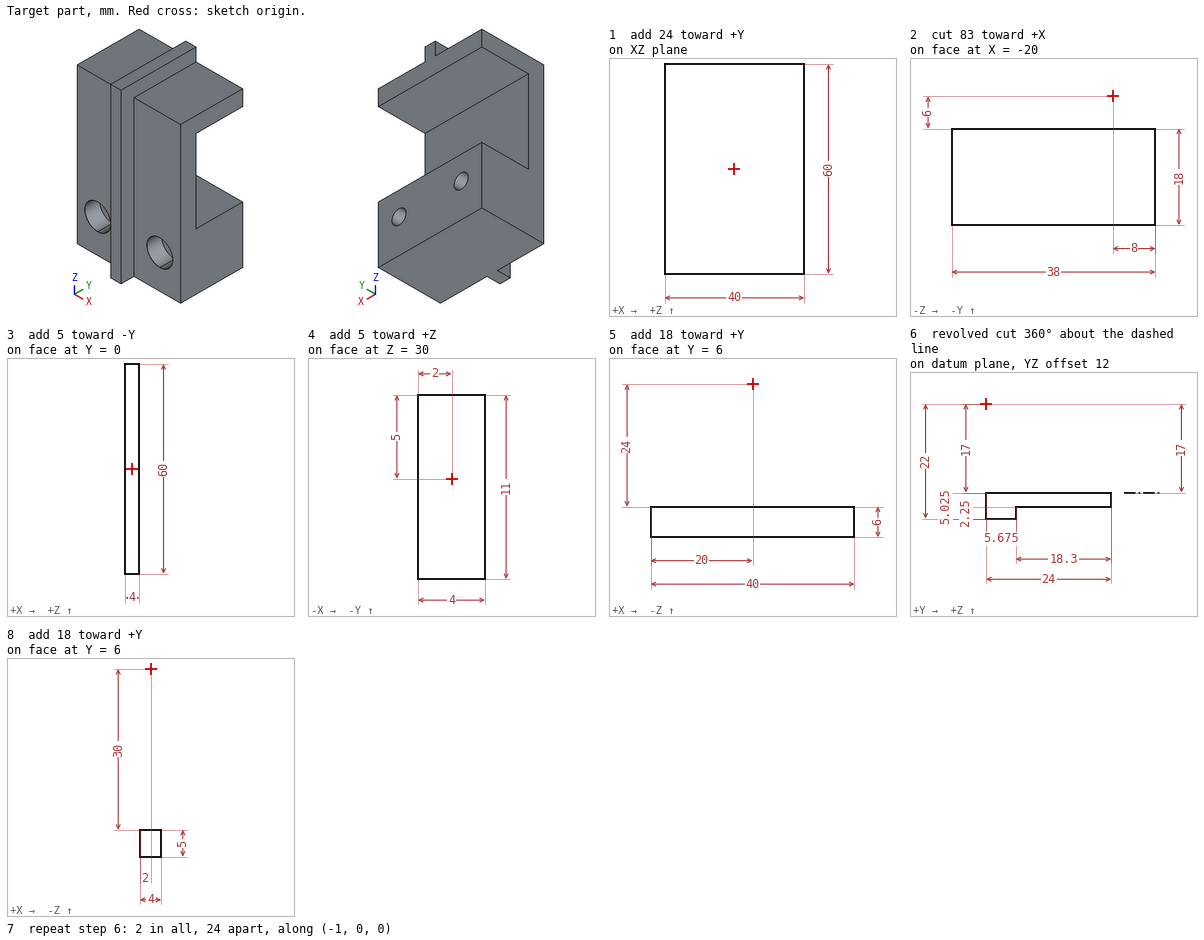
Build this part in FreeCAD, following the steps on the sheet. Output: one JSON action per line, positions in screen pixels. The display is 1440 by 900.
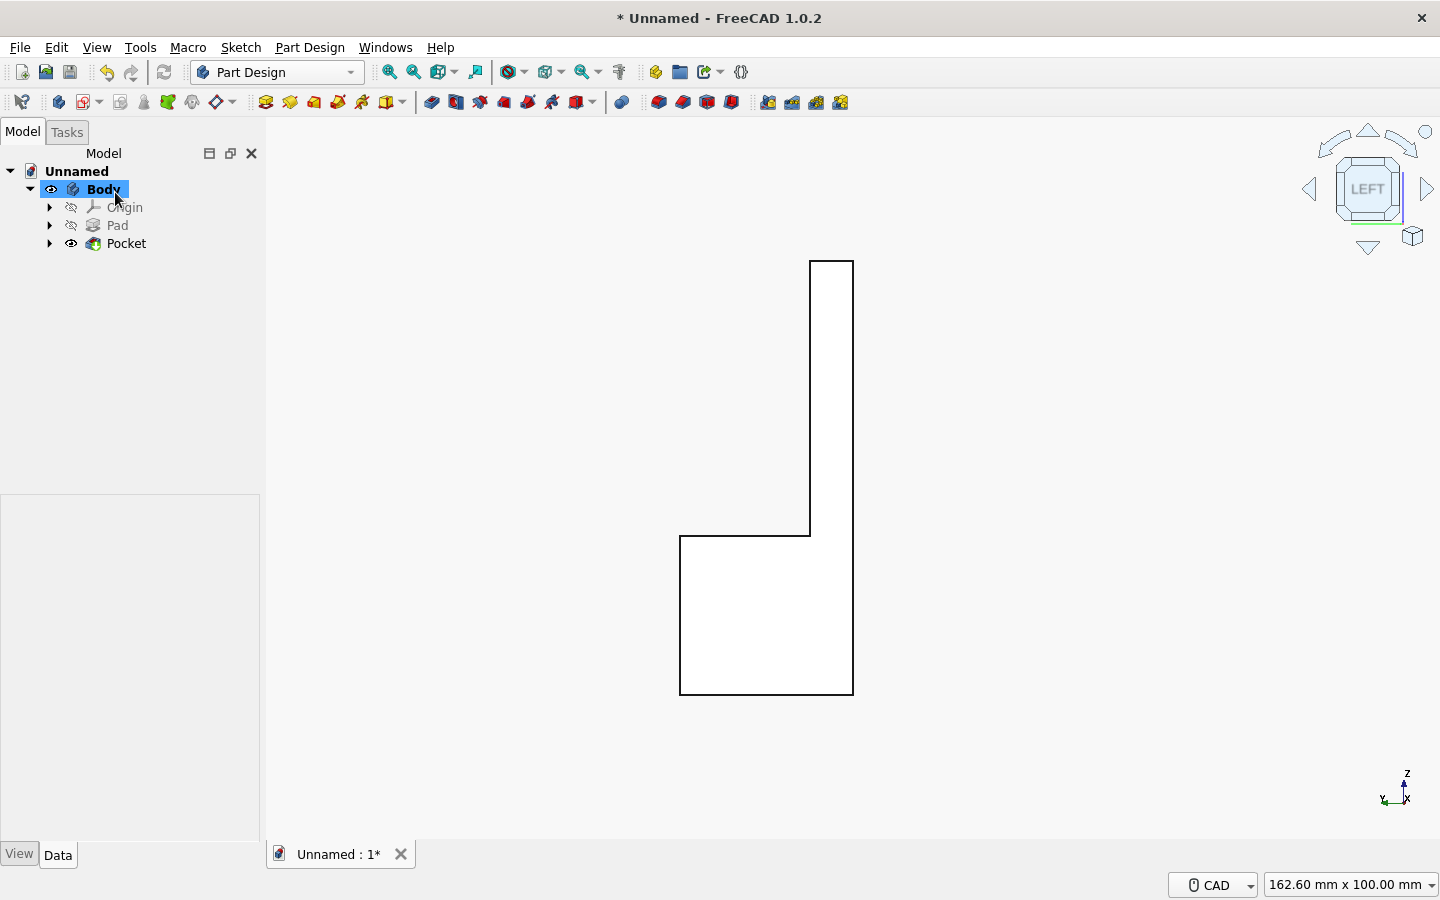
{"action": "key", "text": "0"}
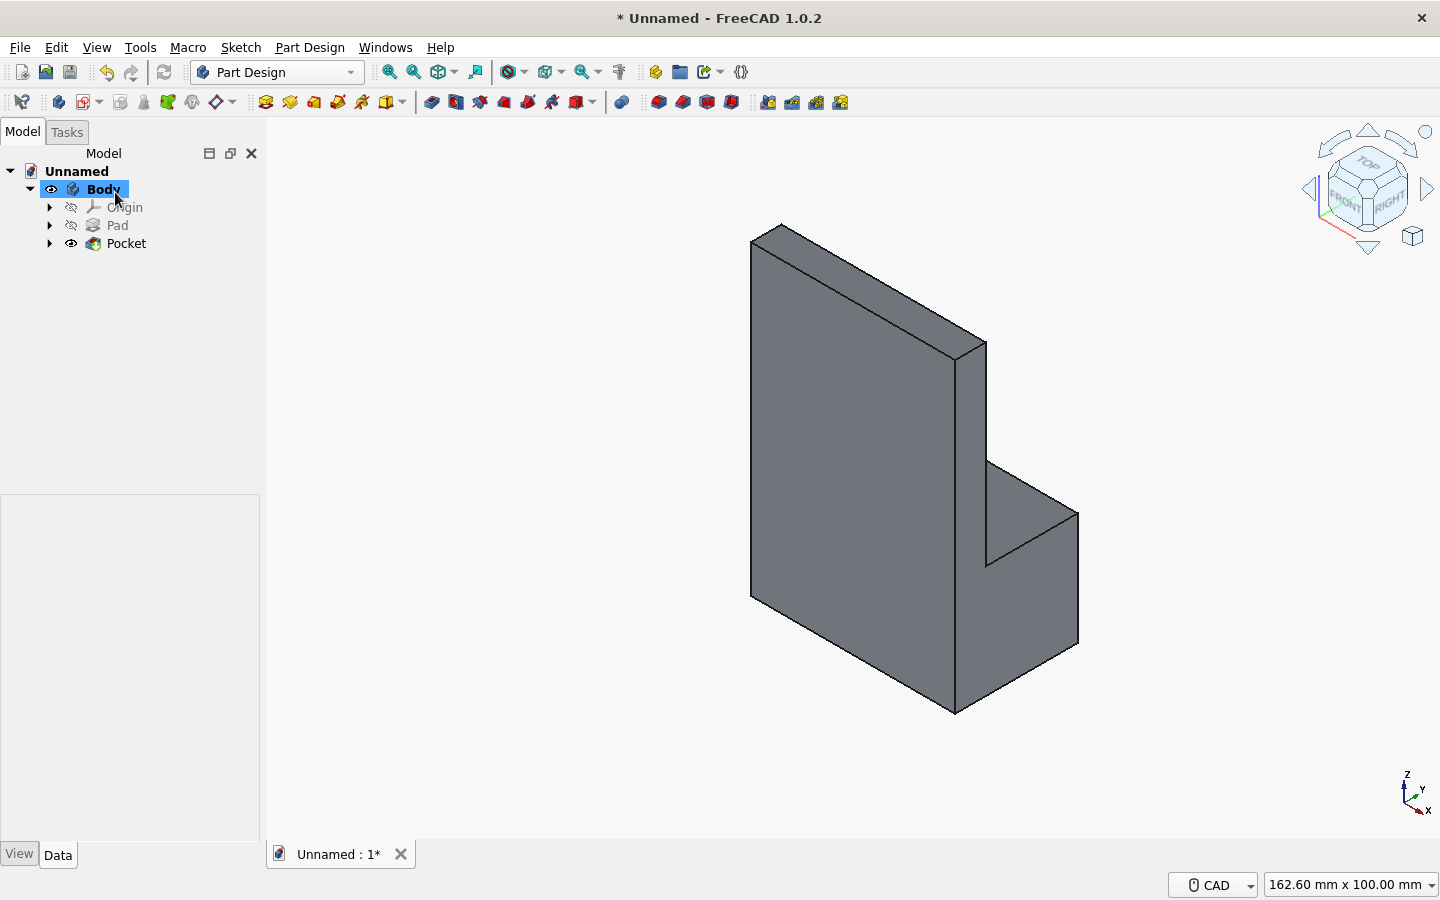
{"action": "left_click", "coordinate": [853, 426]}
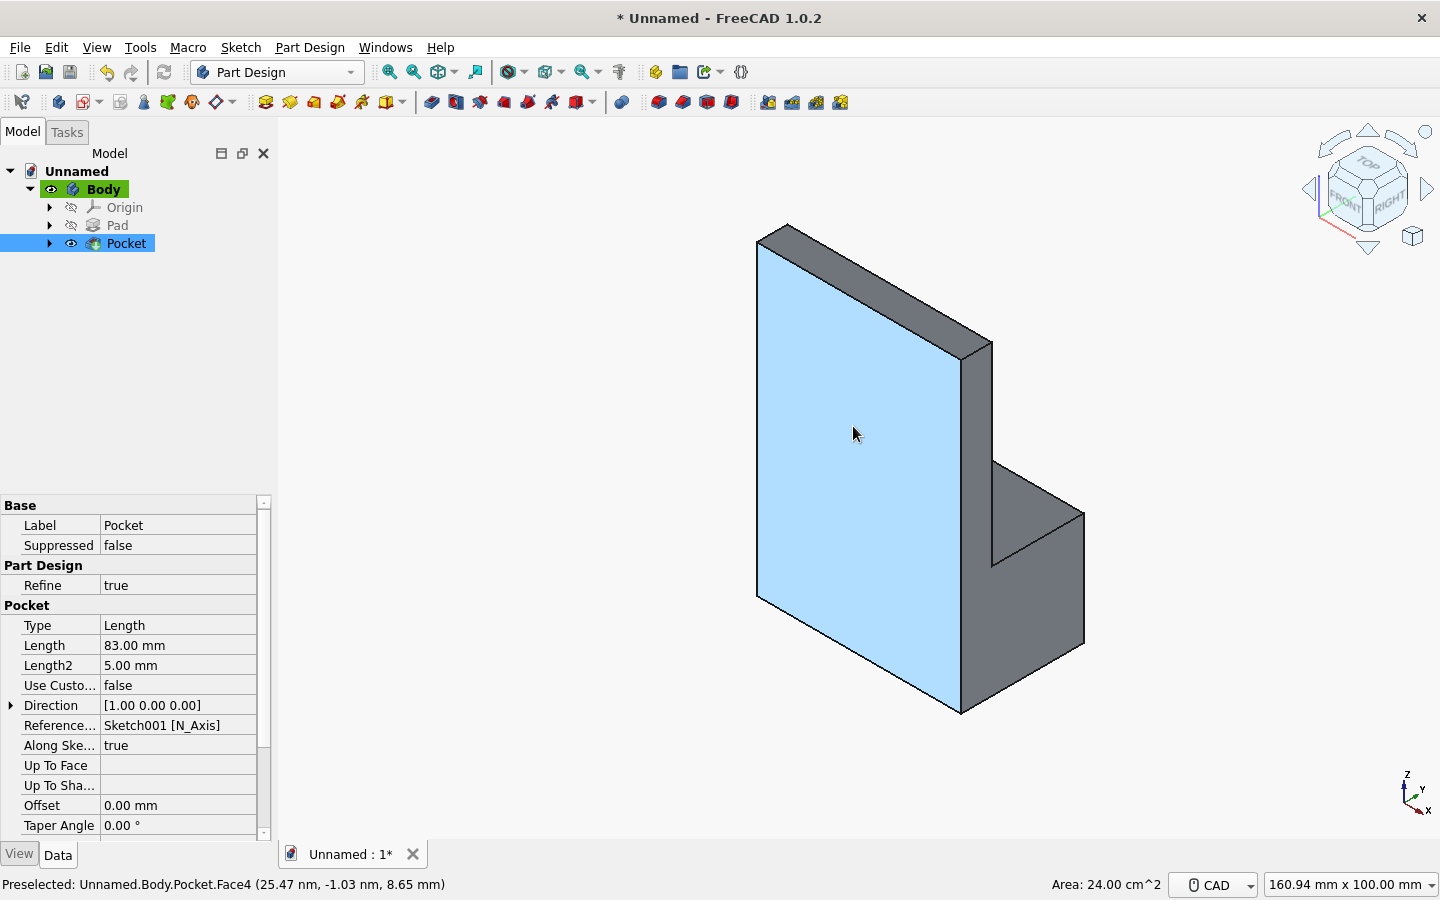
{"action": "left_click", "coordinate": [84, 102]}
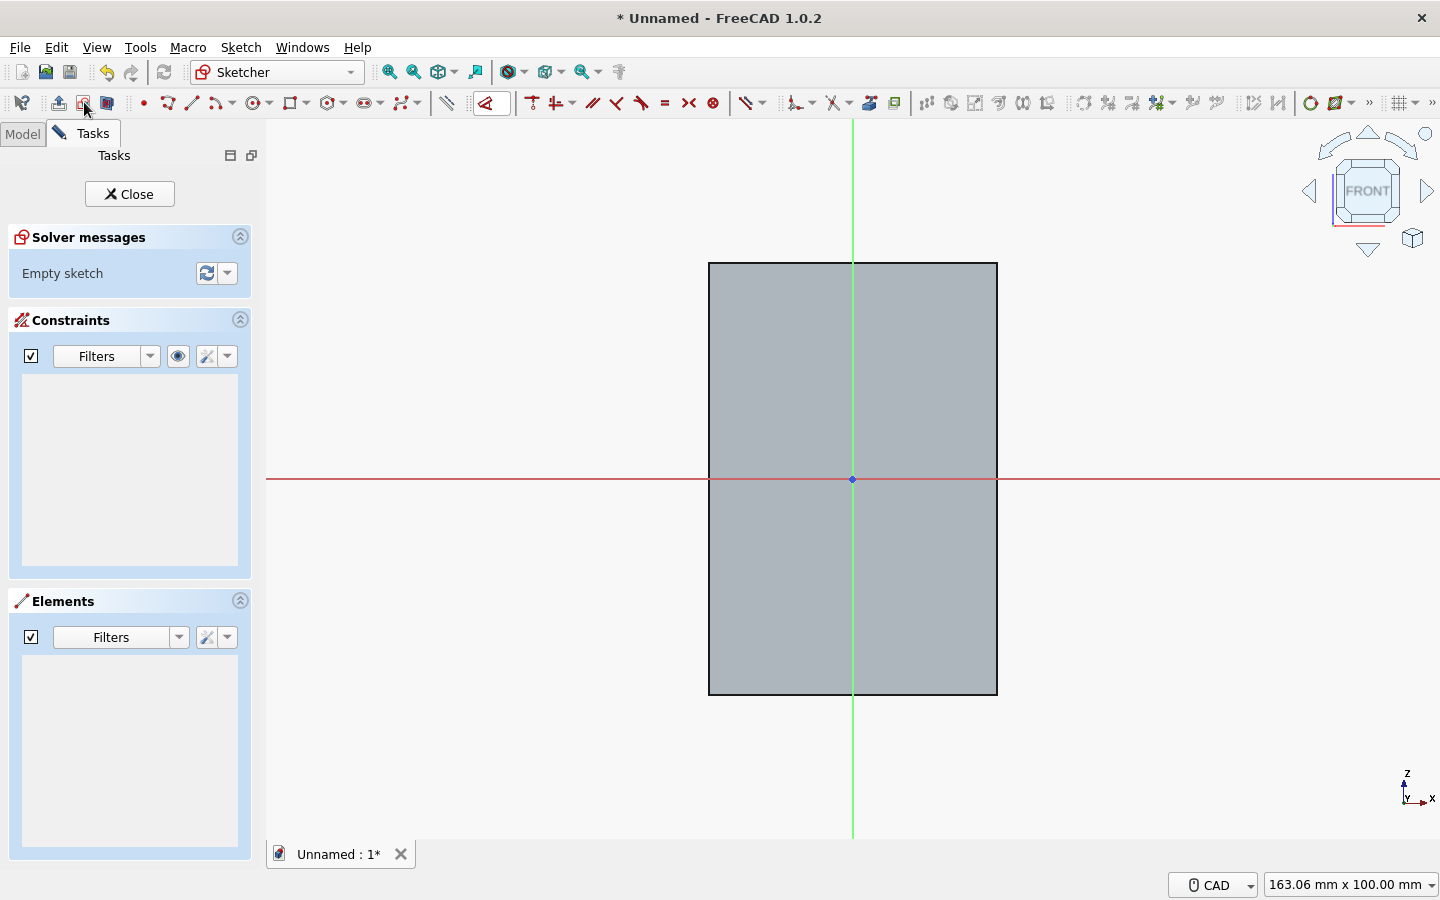
{"action": "key", "text": "g v"}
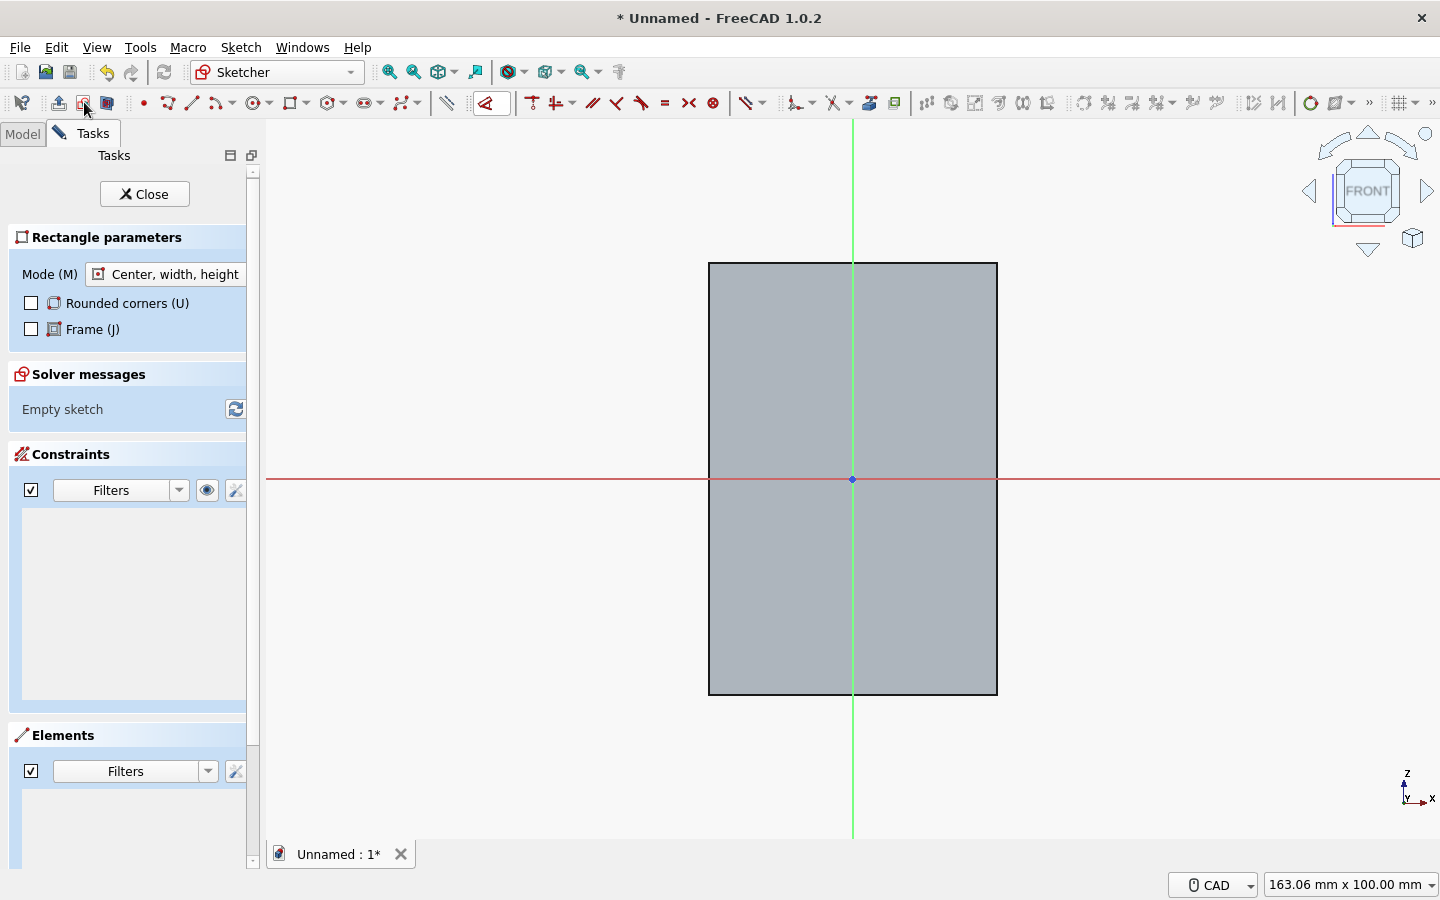
{"action": "left_click", "coordinate": [853, 479]}
{"action": "mouse_move", "coordinate": [867, 263]}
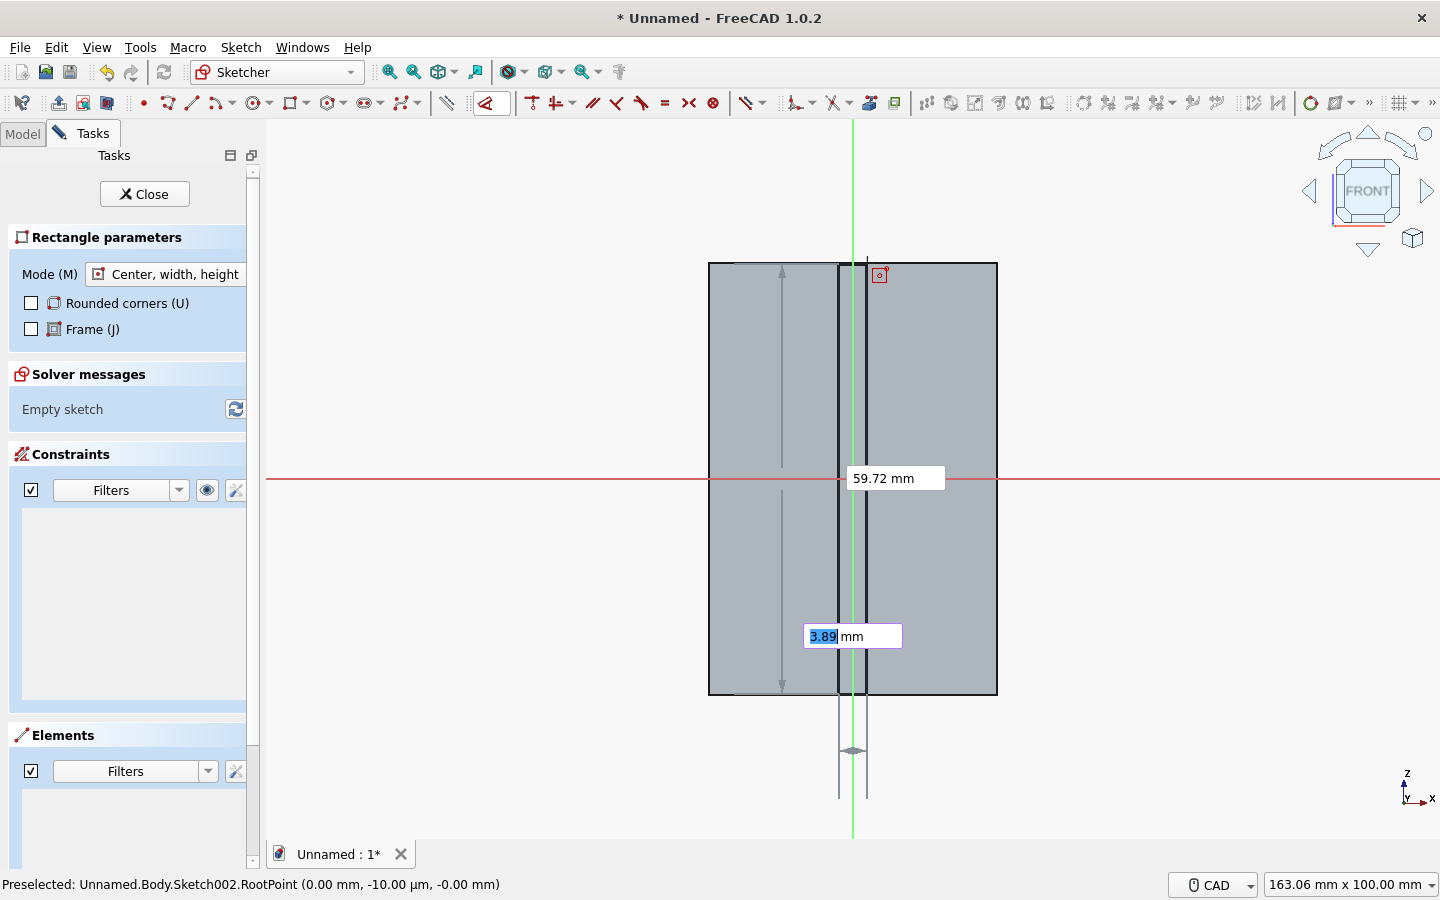
{"action": "type", "text": "4"}
{"action": "key", "text": "Tab"}
{"action": "type", "text": "60"}
{"action": "key", "text": "Return"}
{"action": "key", "text": "Escape"}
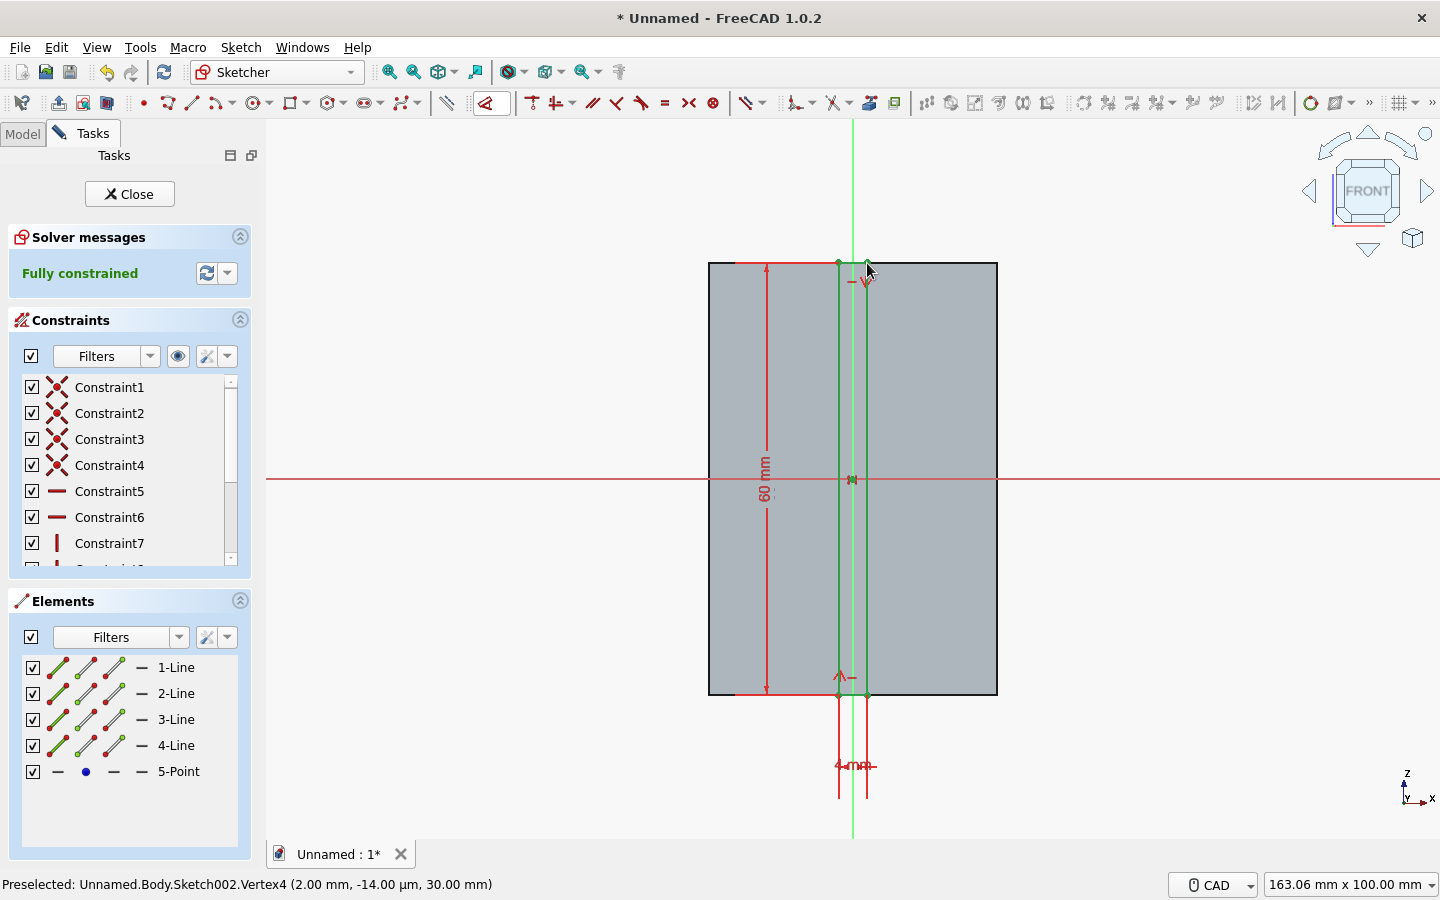
{"action": "left_click", "coordinate": [130, 194]}